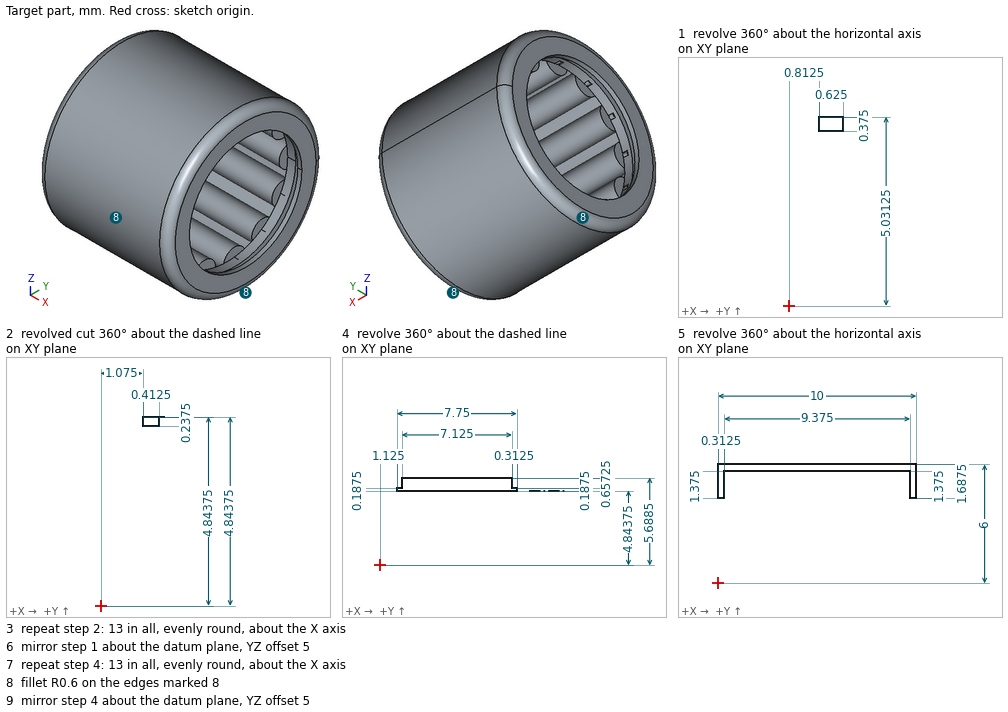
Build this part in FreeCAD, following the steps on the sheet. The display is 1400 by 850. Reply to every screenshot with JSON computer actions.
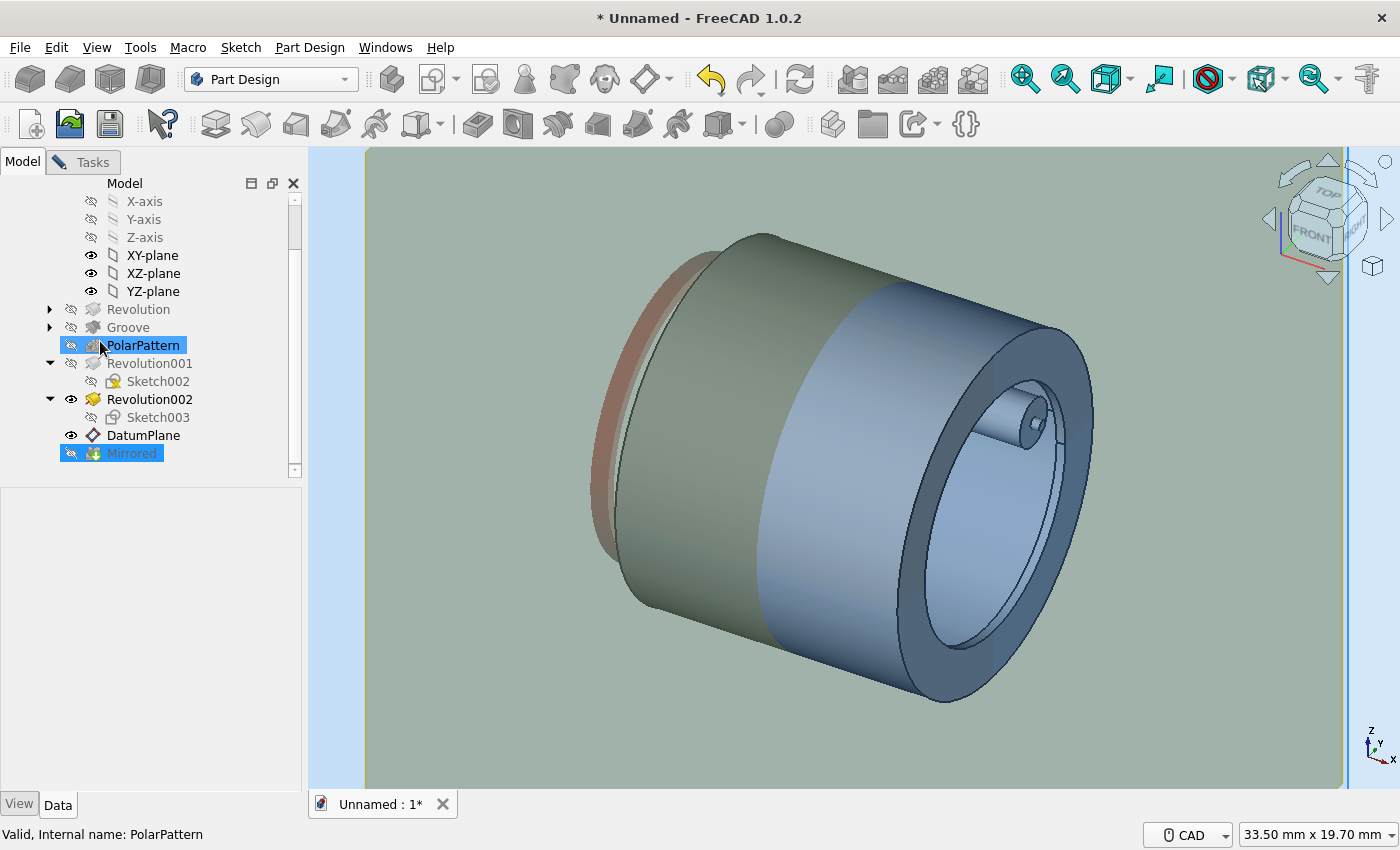
{"action": "left_click", "coordinate": [116, 435]}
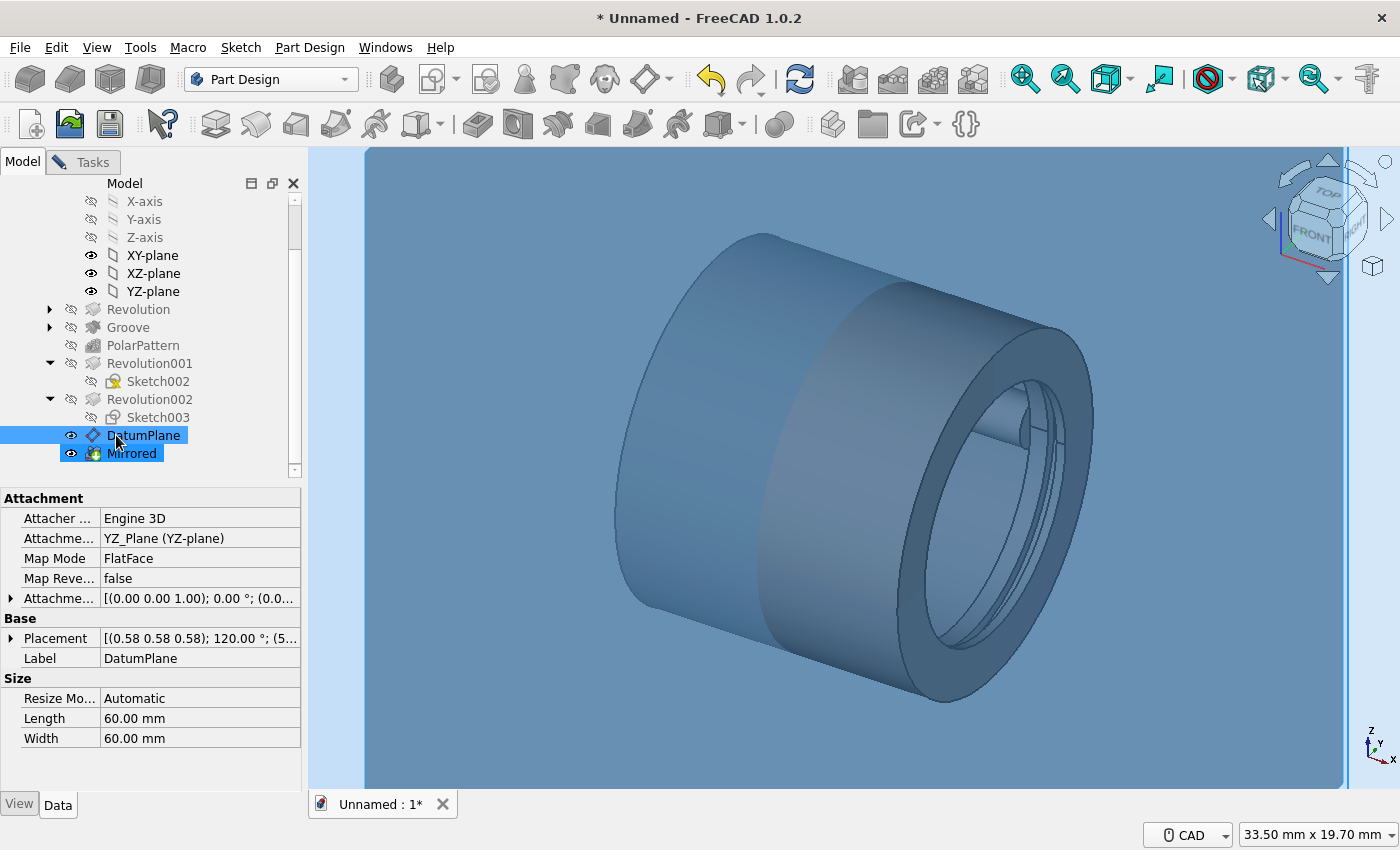
{"action": "left_click", "coordinate": [84, 161]}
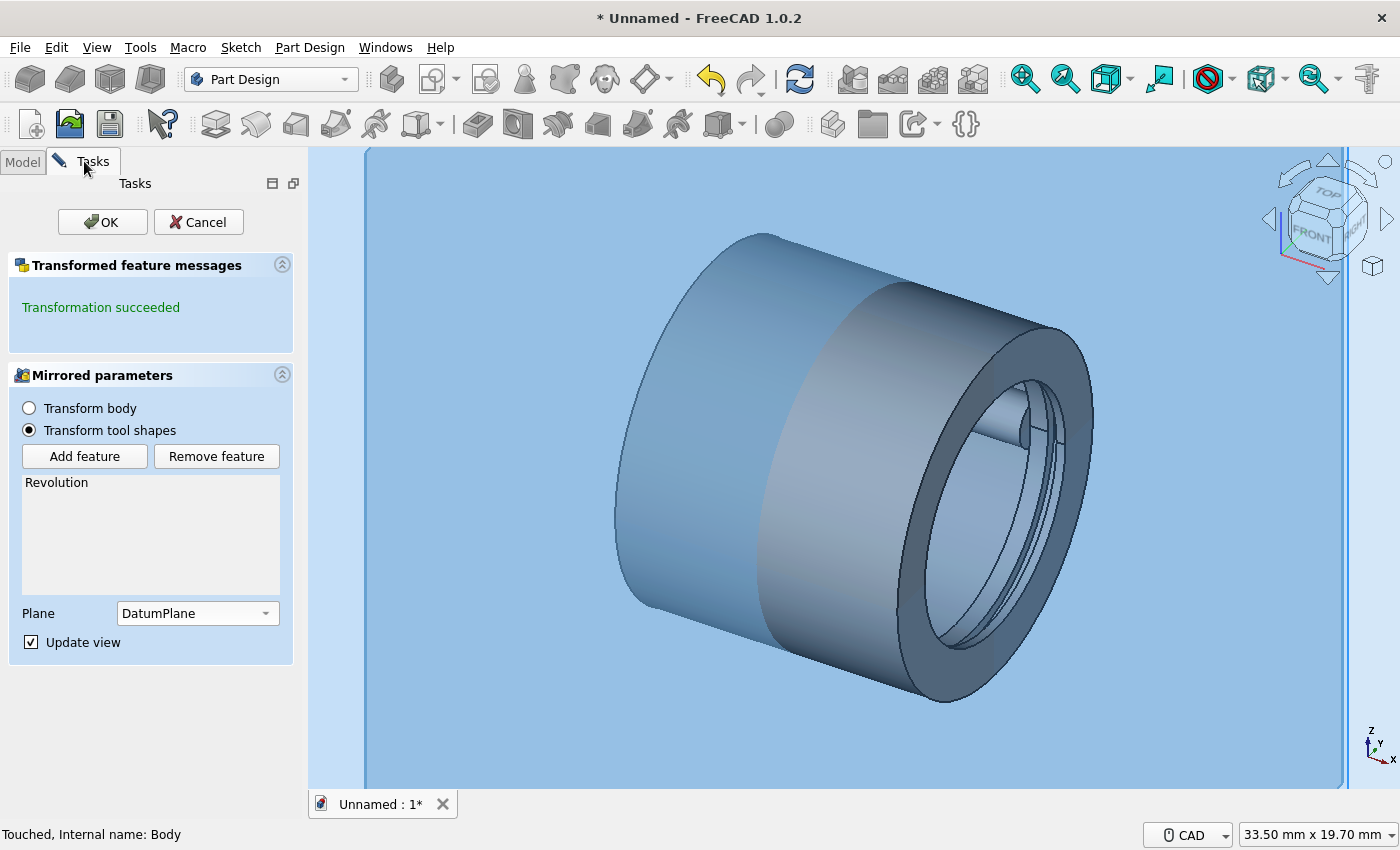
{"action": "left_click", "coordinate": [103, 222]}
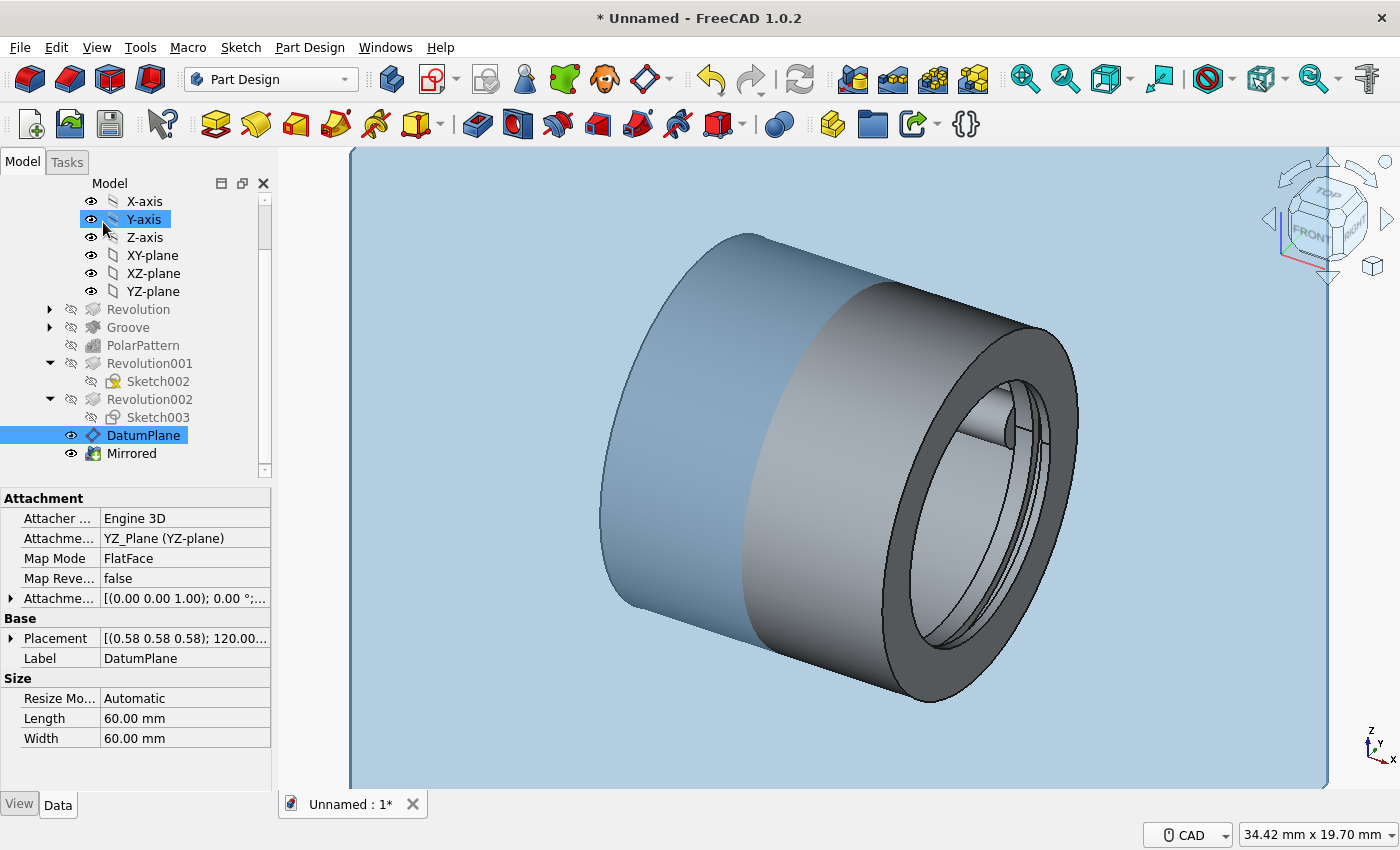
{"action": "left_click", "coordinate": [116, 435]}
{"action": "key", "text": "space"}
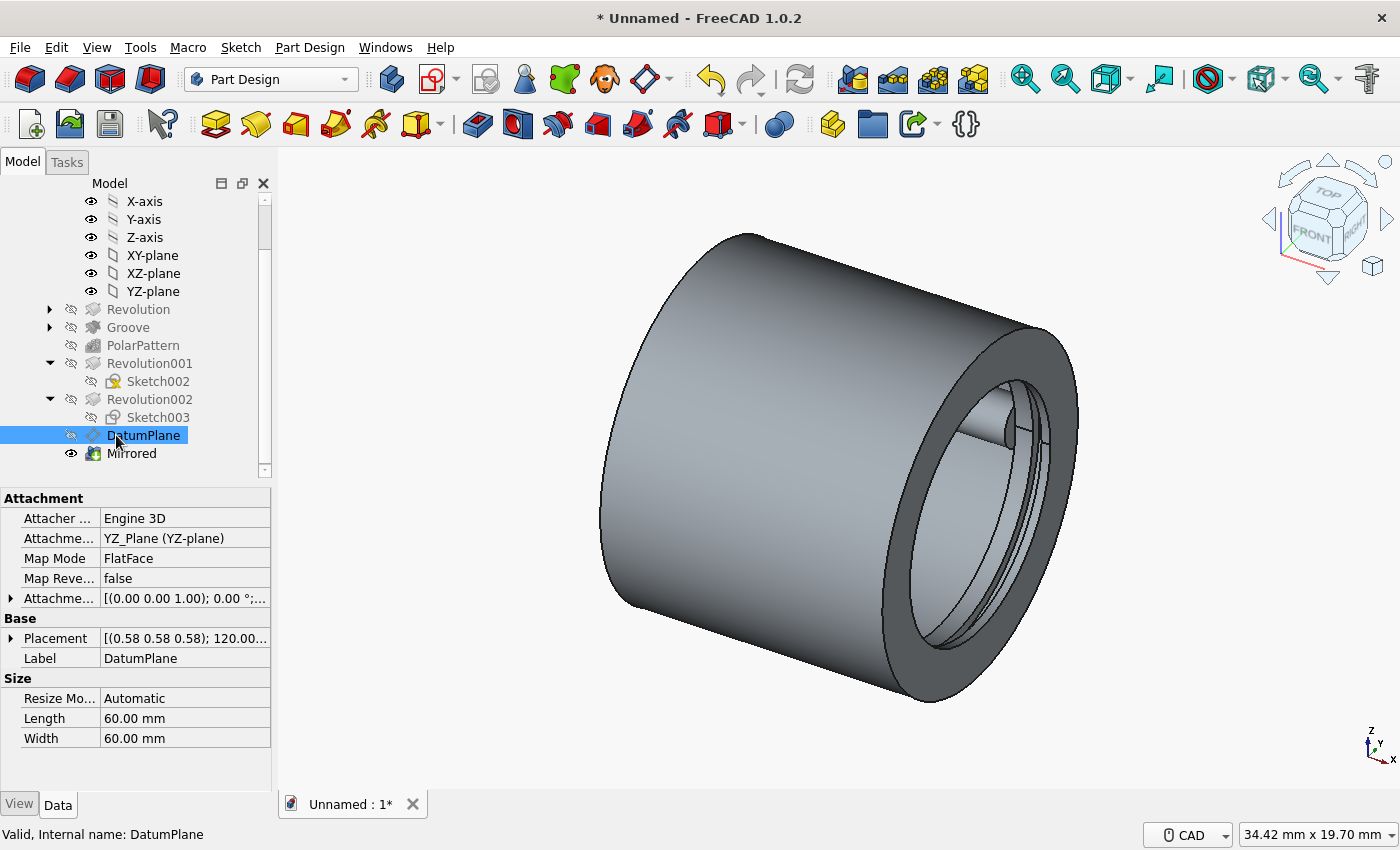
{"action": "left_click", "coordinate": [116, 363]}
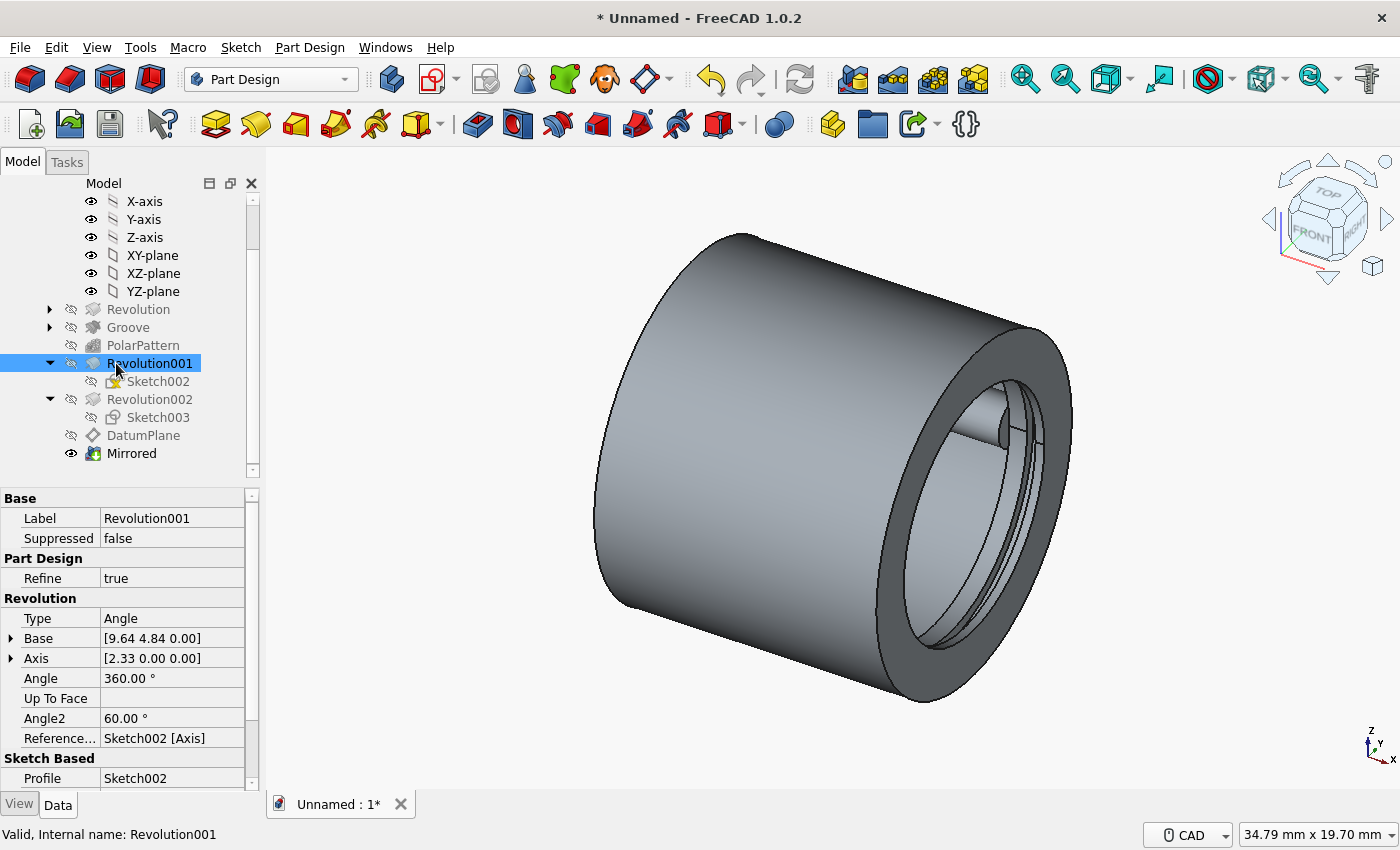
{"action": "left_click", "coordinate": [934, 80]}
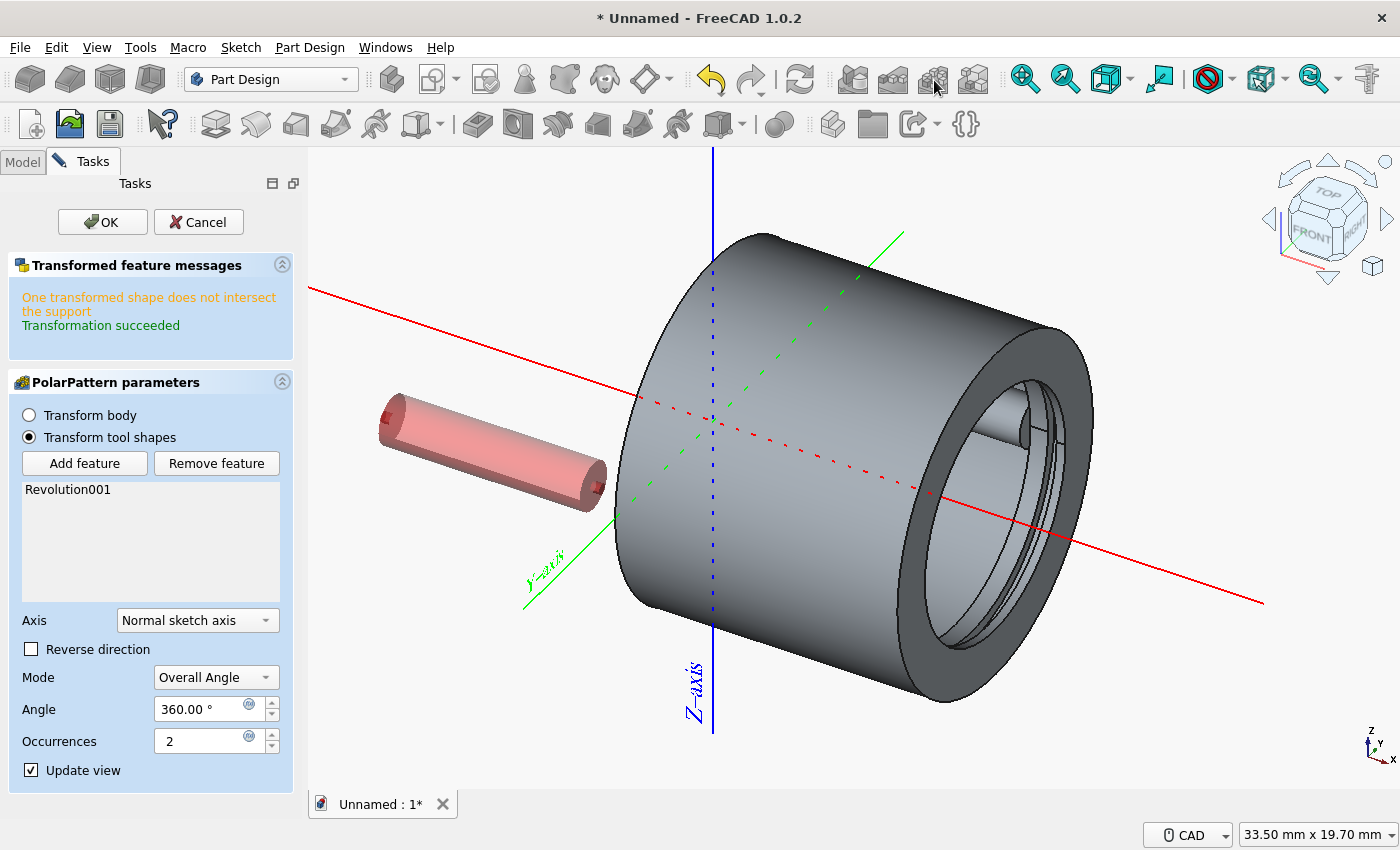
{"action": "left_click", "coordinate": [198, 620]}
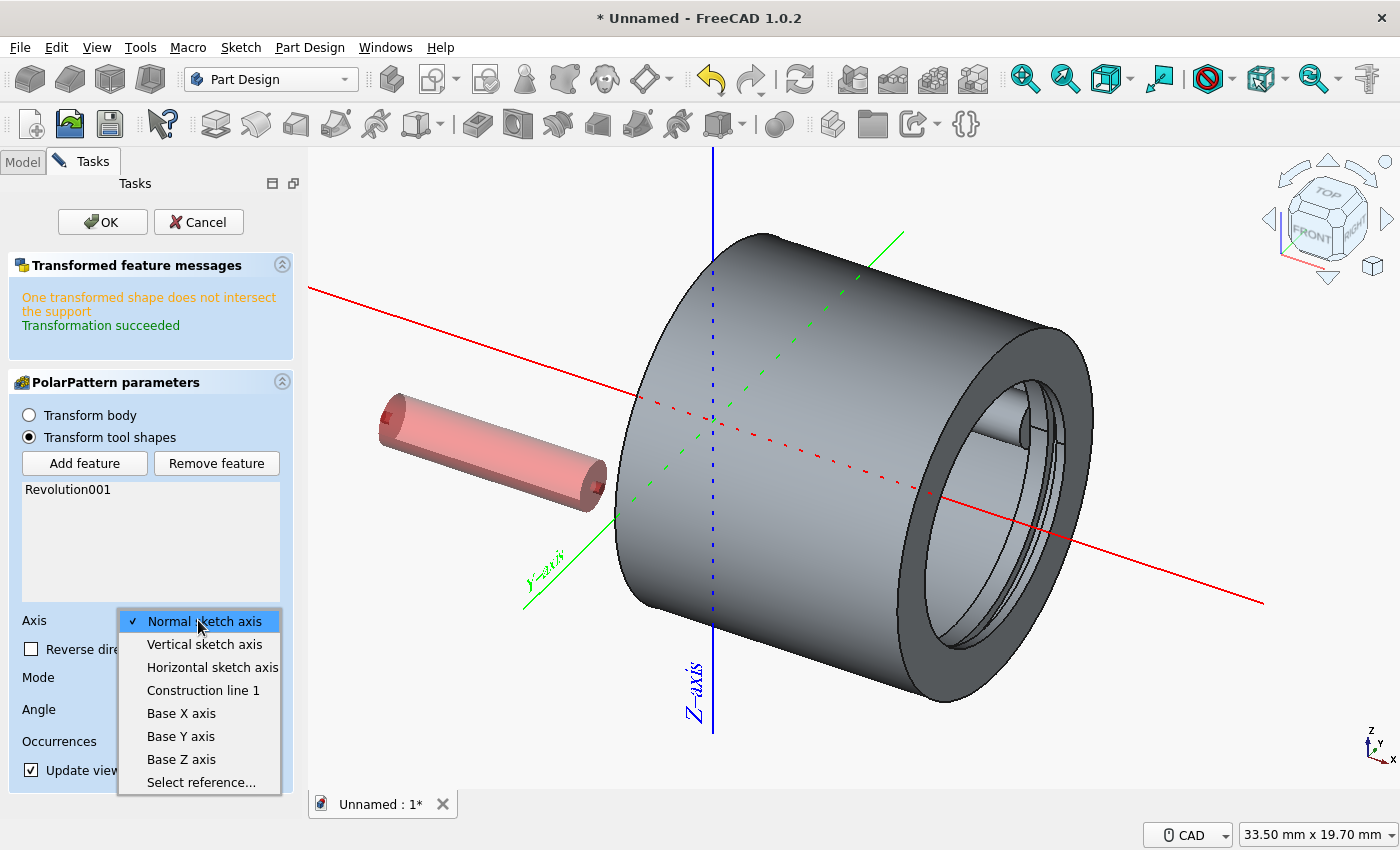
{"action": "left_click", "coordinate": [198, 714]}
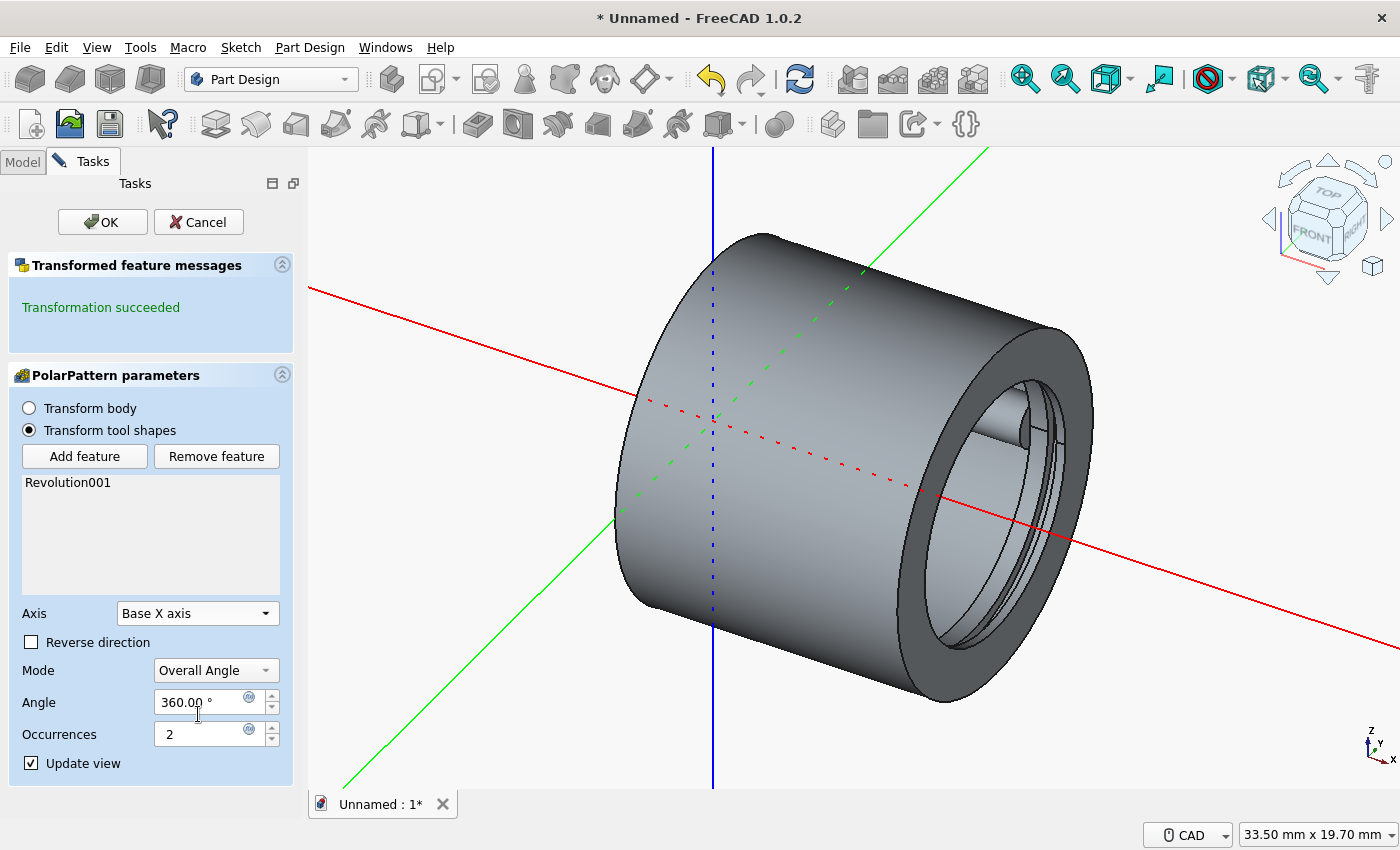
{"action": "triple_click", "coordinate": [209, 734]}